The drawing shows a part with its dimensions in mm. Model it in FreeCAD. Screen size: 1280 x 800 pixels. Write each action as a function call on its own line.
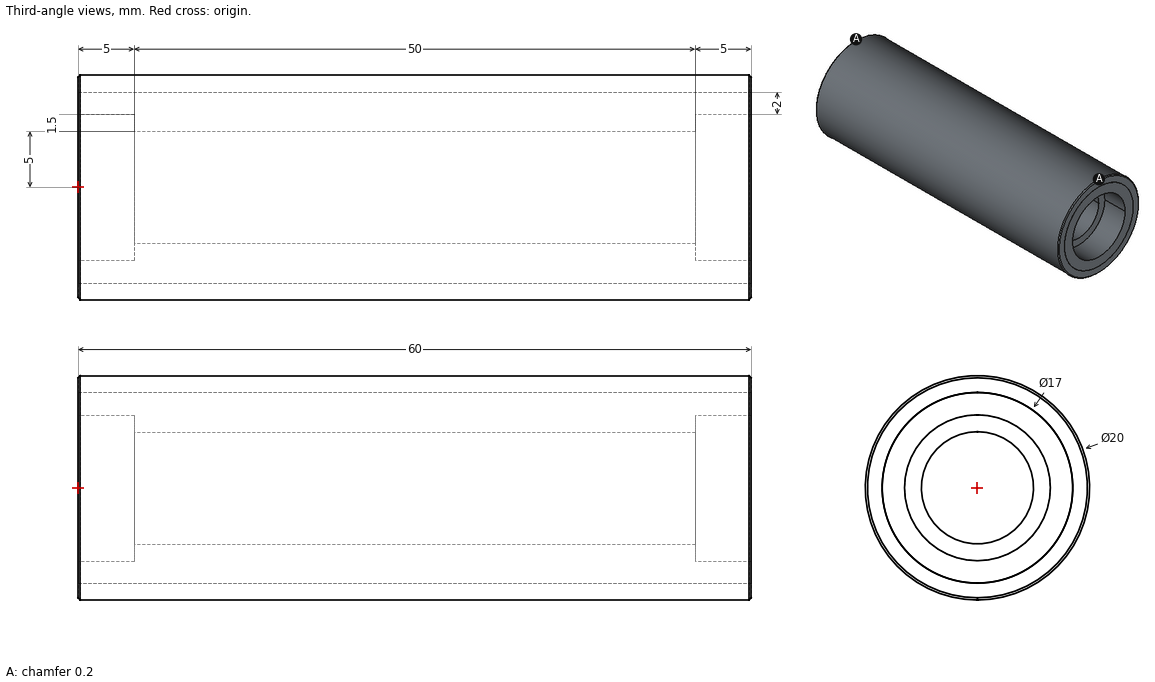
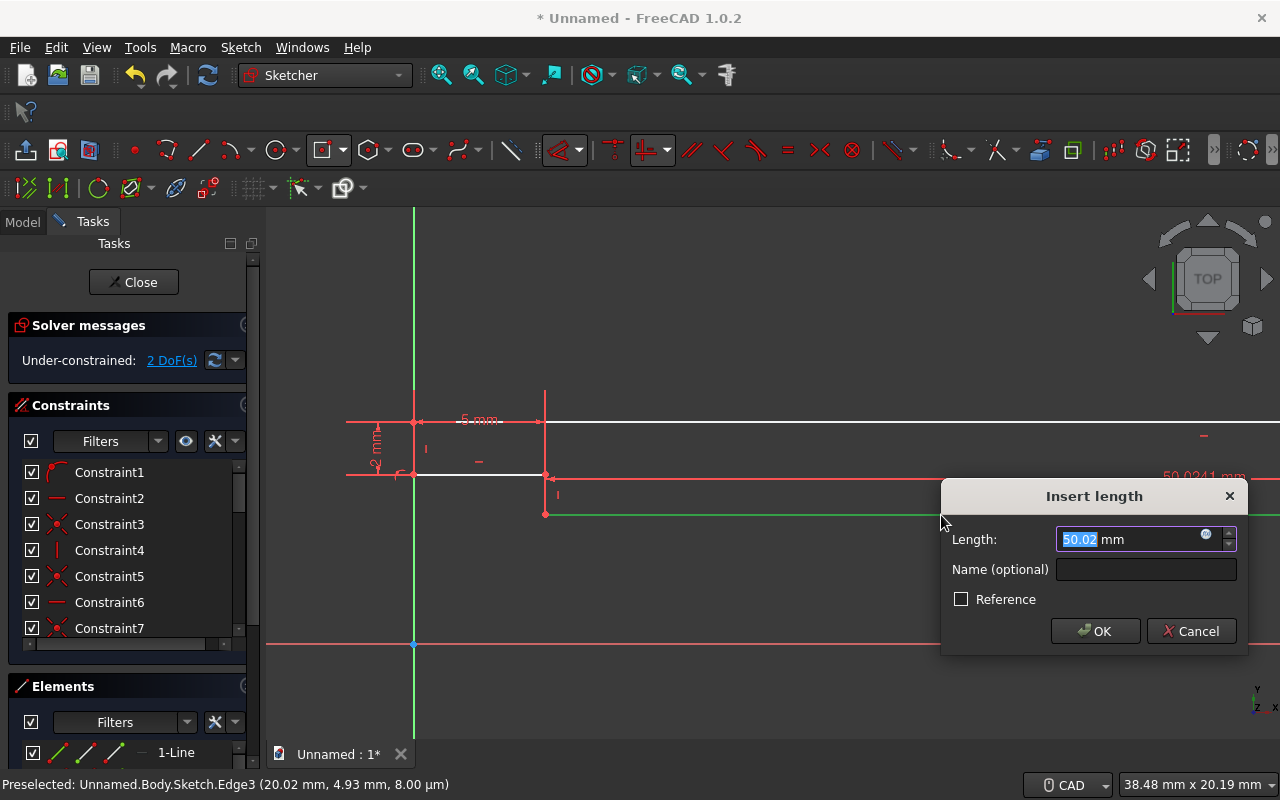
text(50)
key(Return)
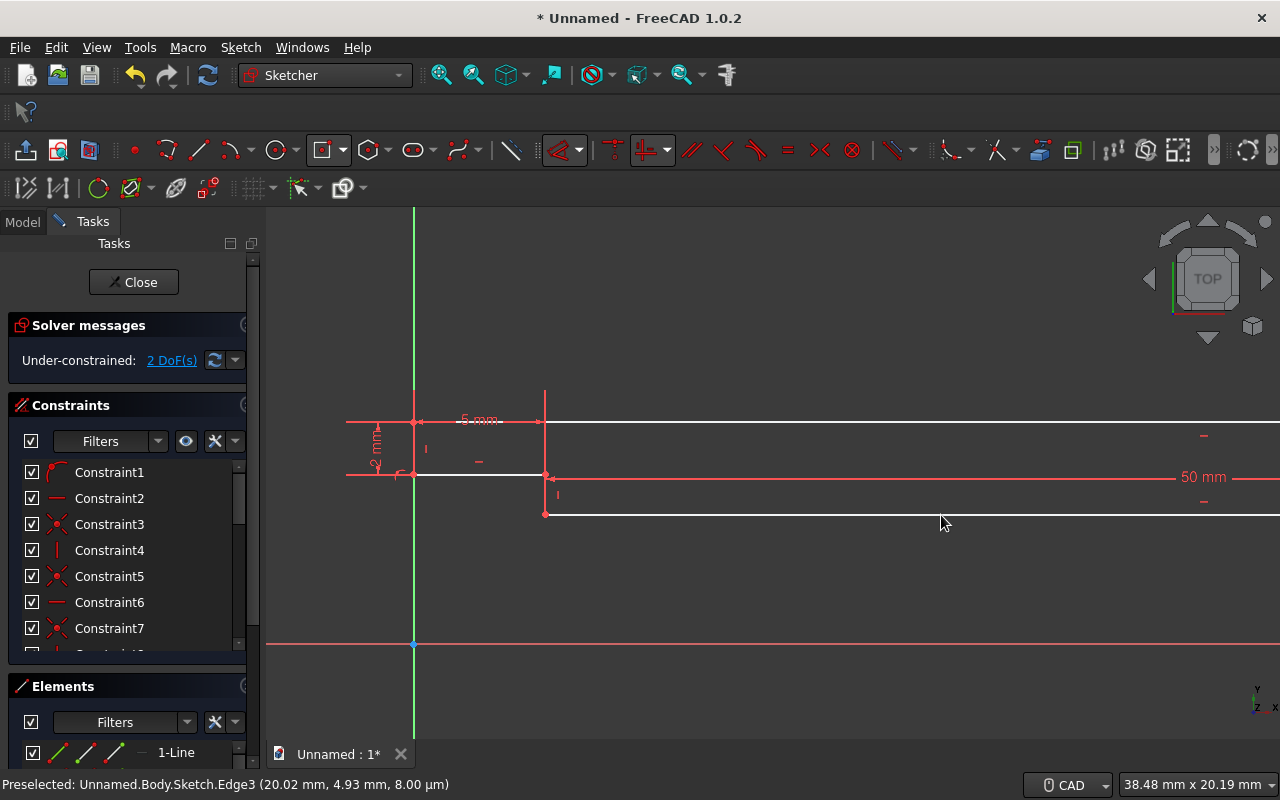
click(545, 515)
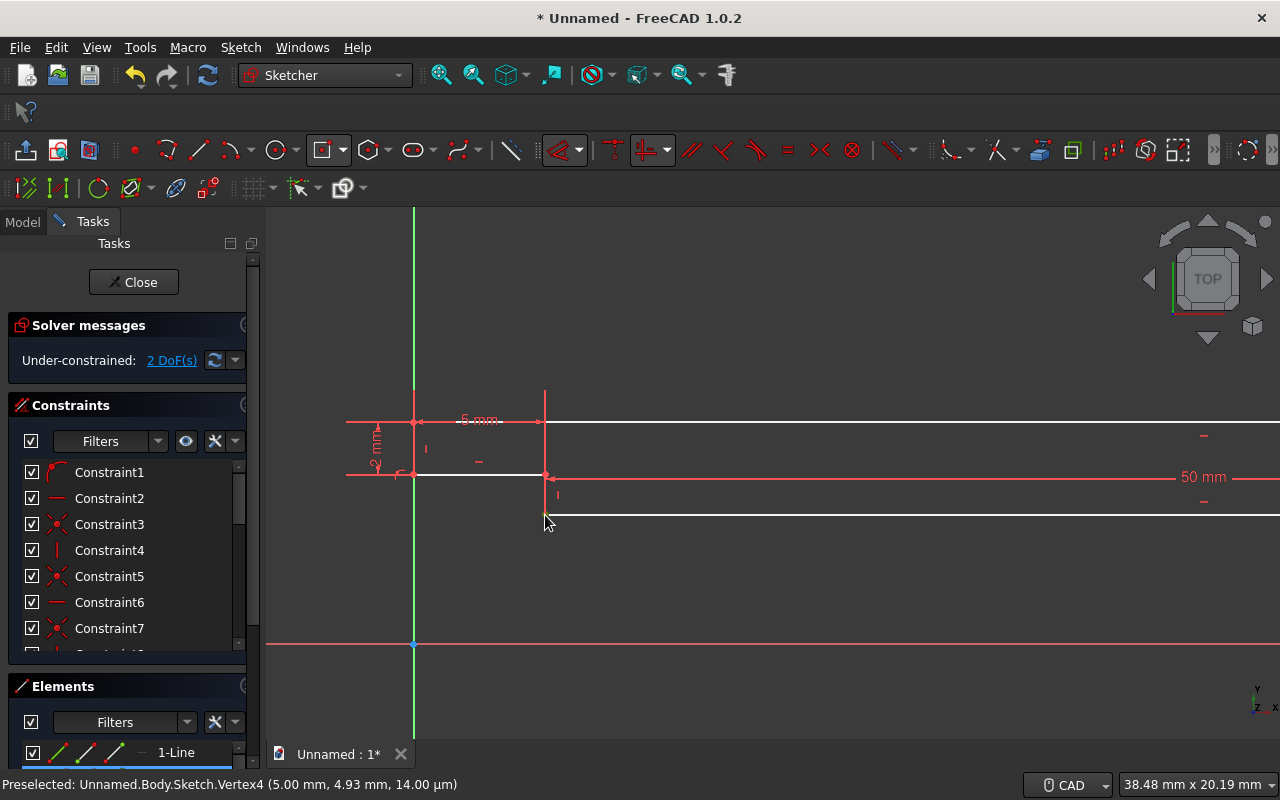
key(i)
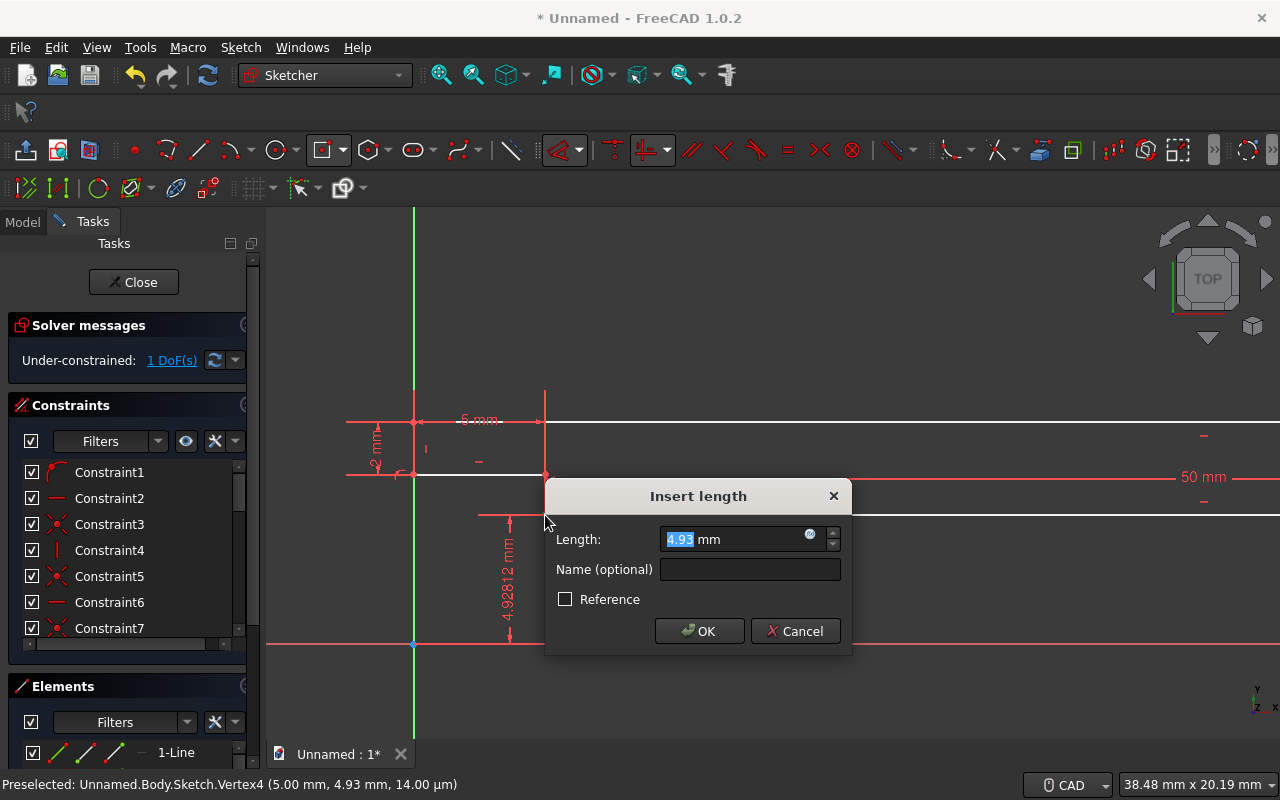
text(5)
key(Return)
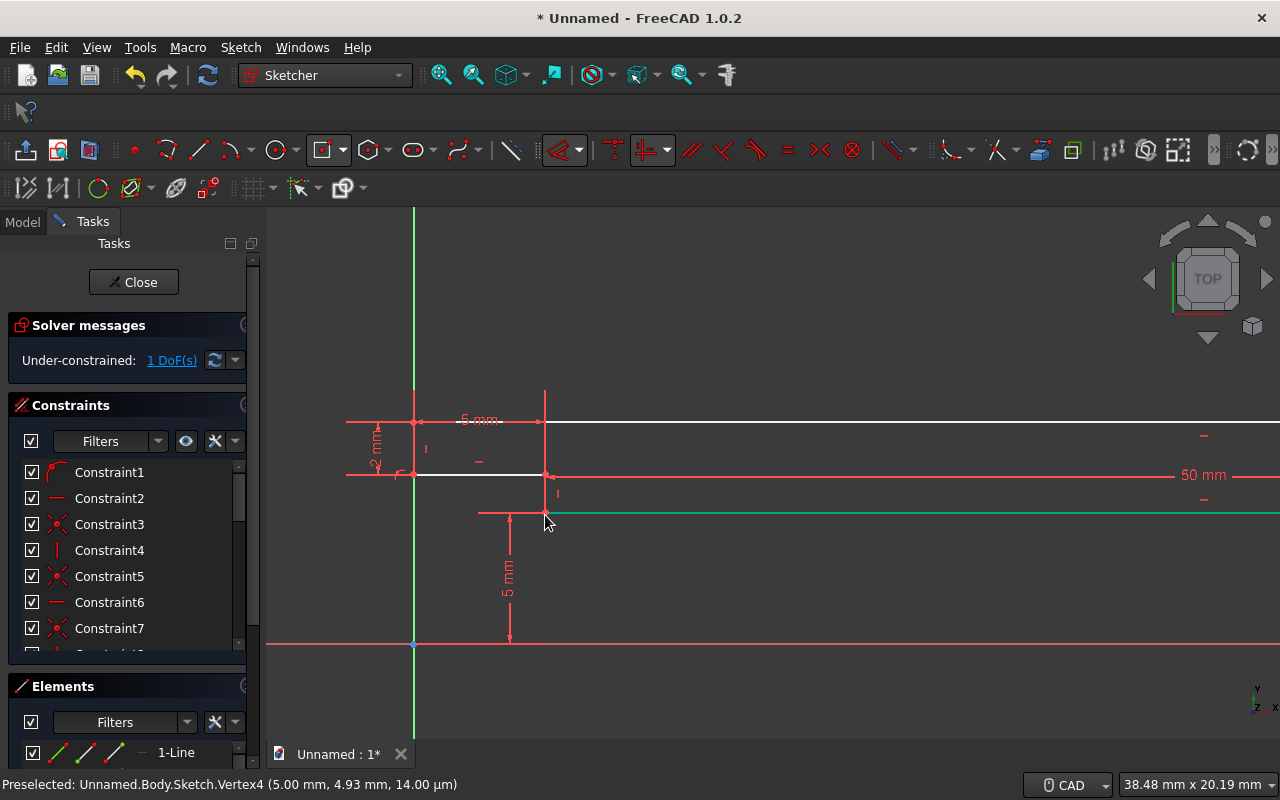
click(545, 486)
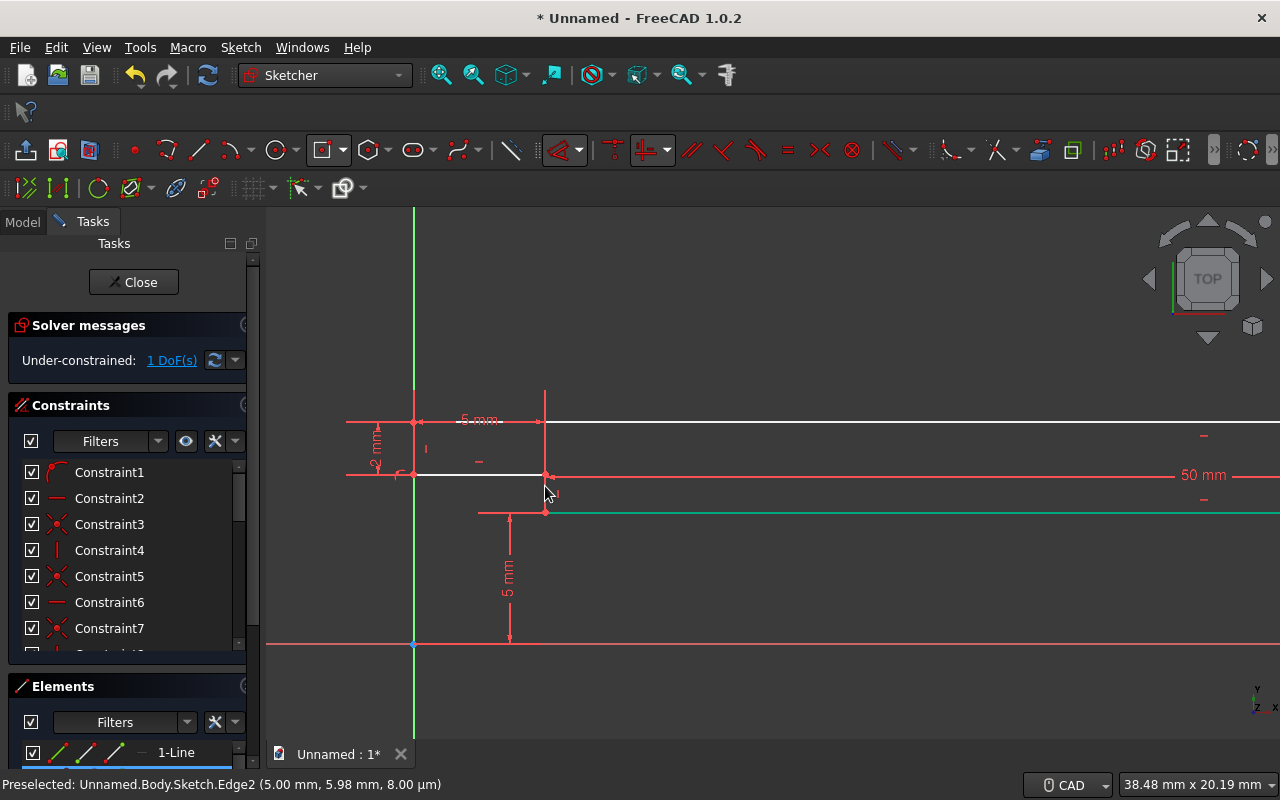
key(i)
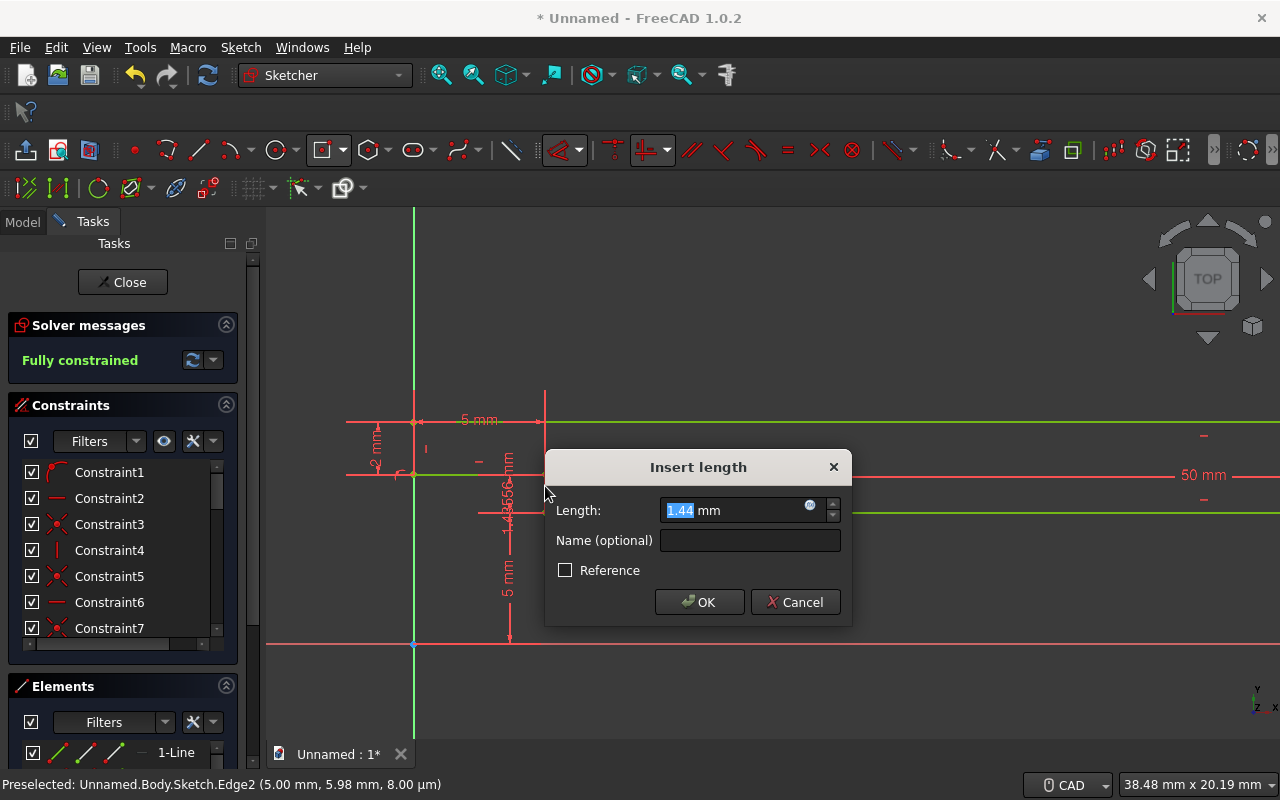
text(1.5)
key(Return)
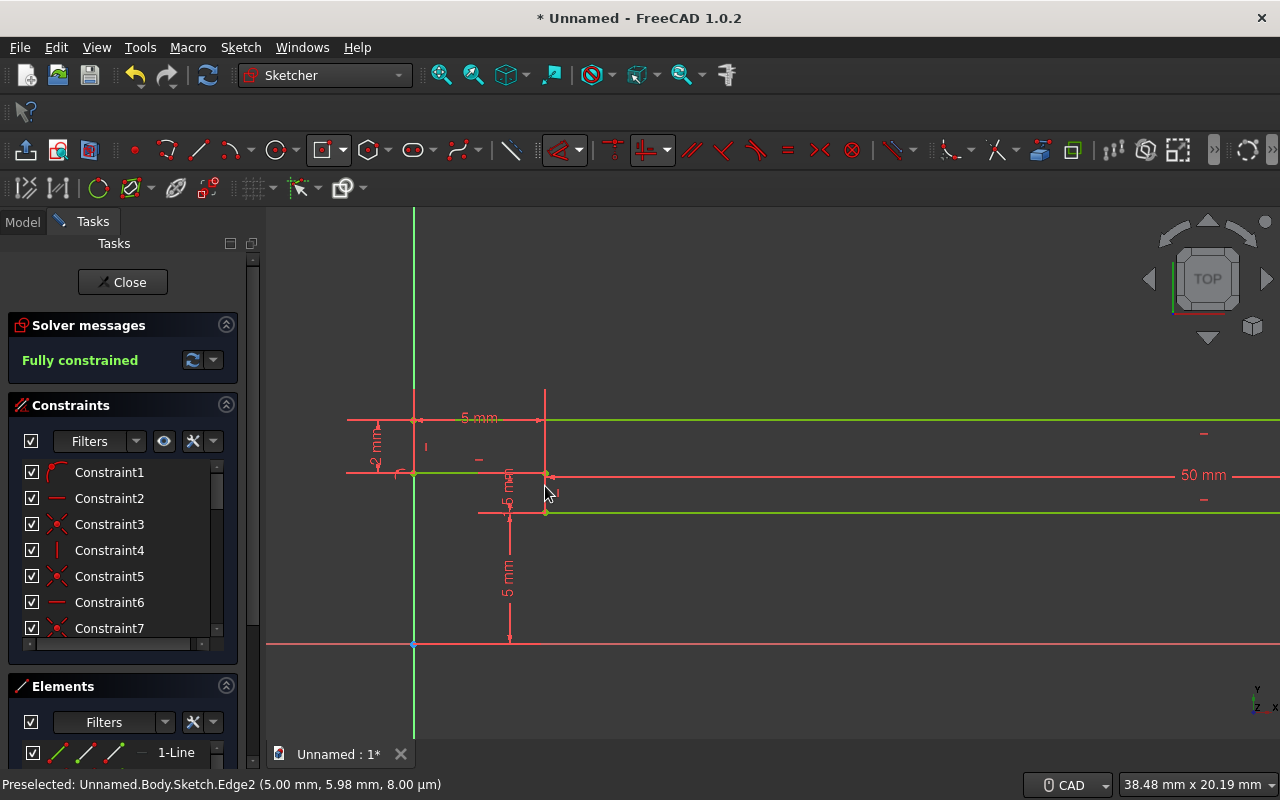
click(123, 282)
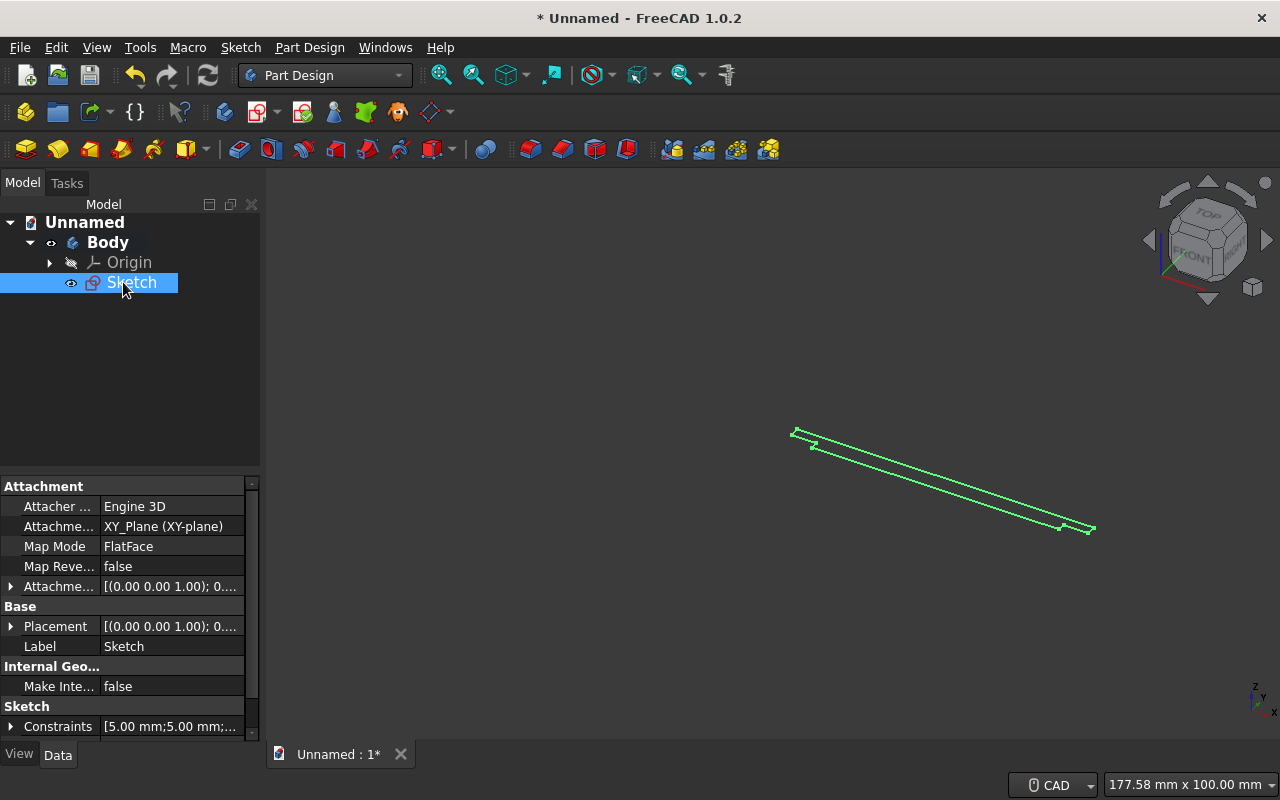
click(58, 150)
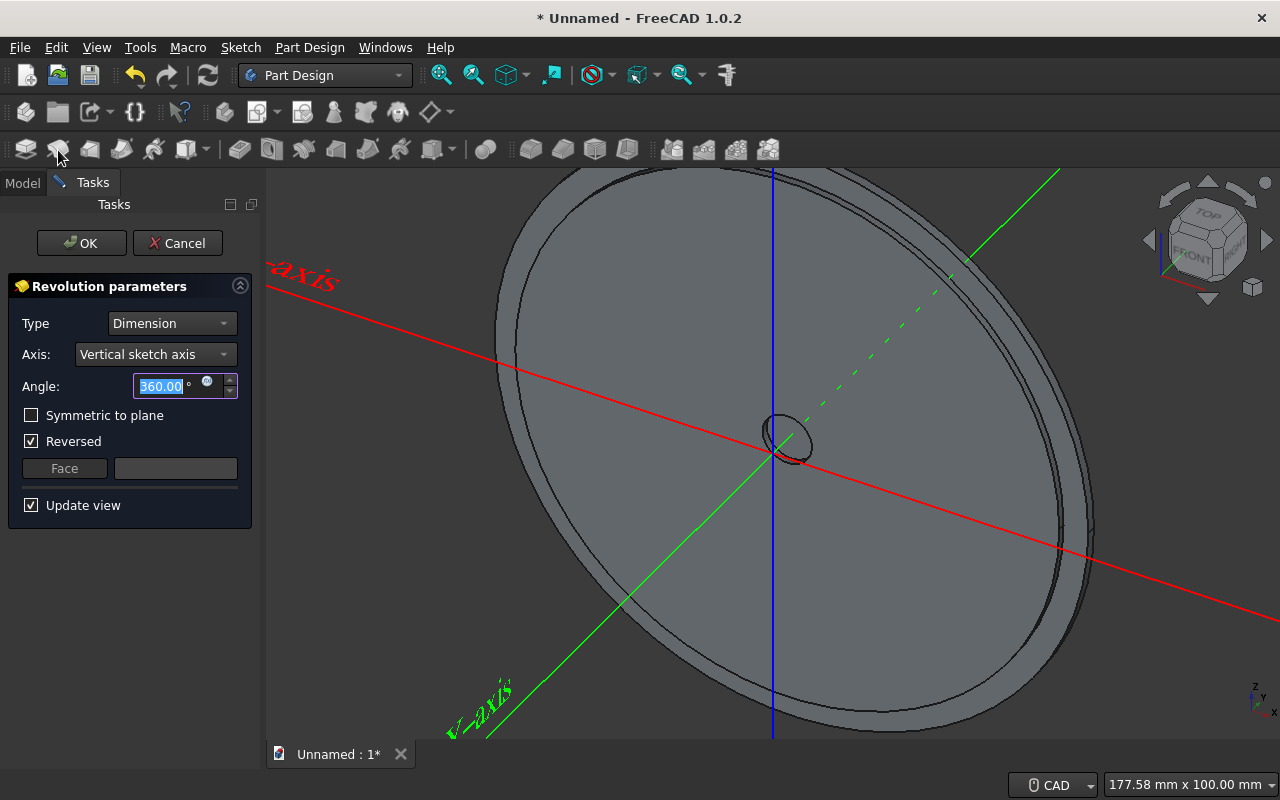
click(156, 354)